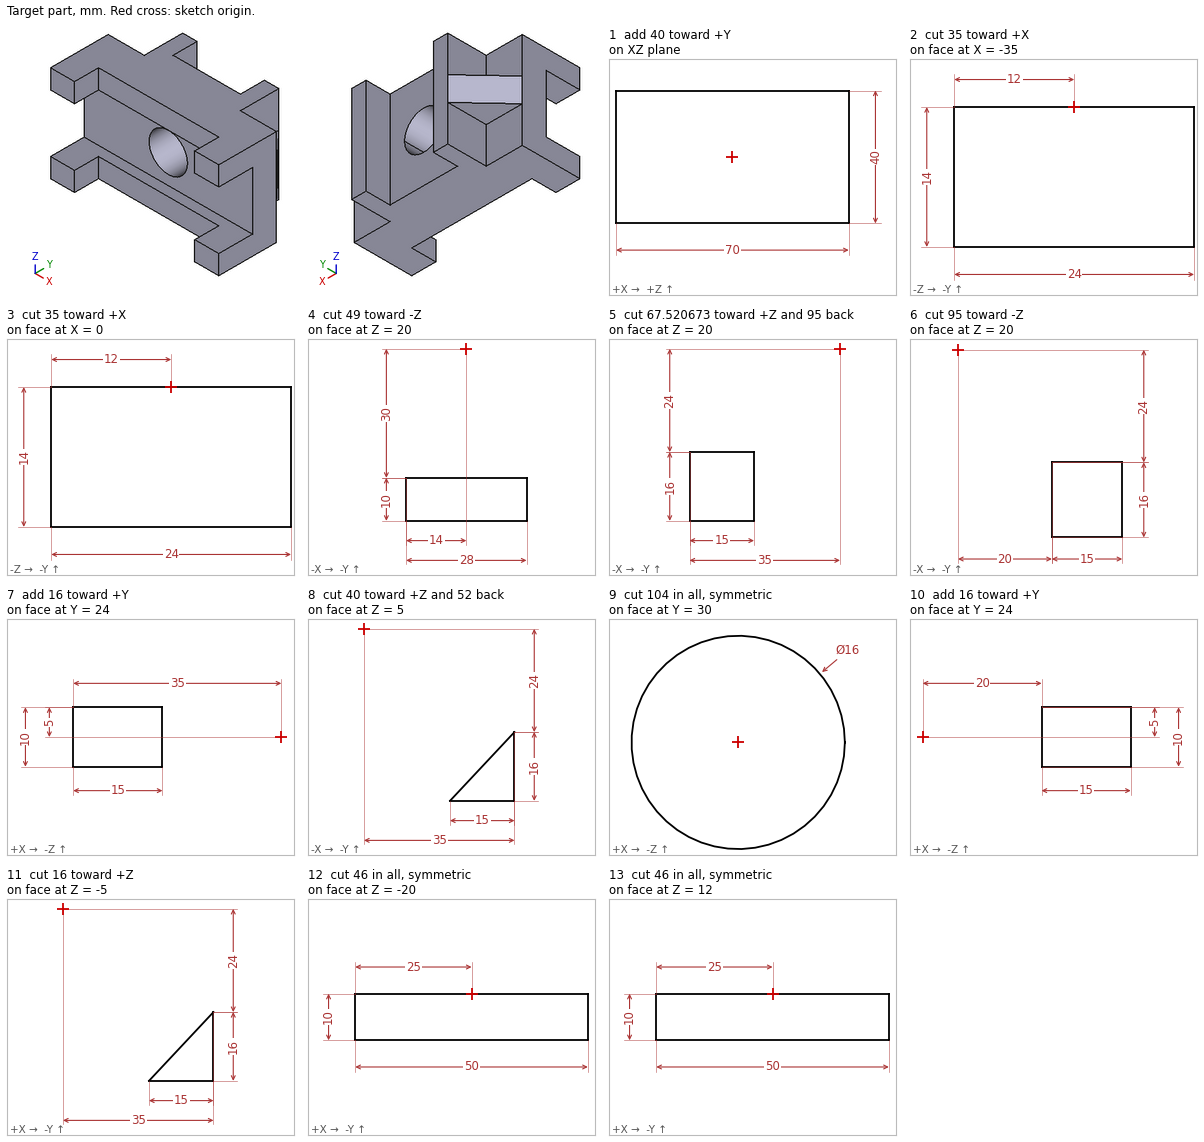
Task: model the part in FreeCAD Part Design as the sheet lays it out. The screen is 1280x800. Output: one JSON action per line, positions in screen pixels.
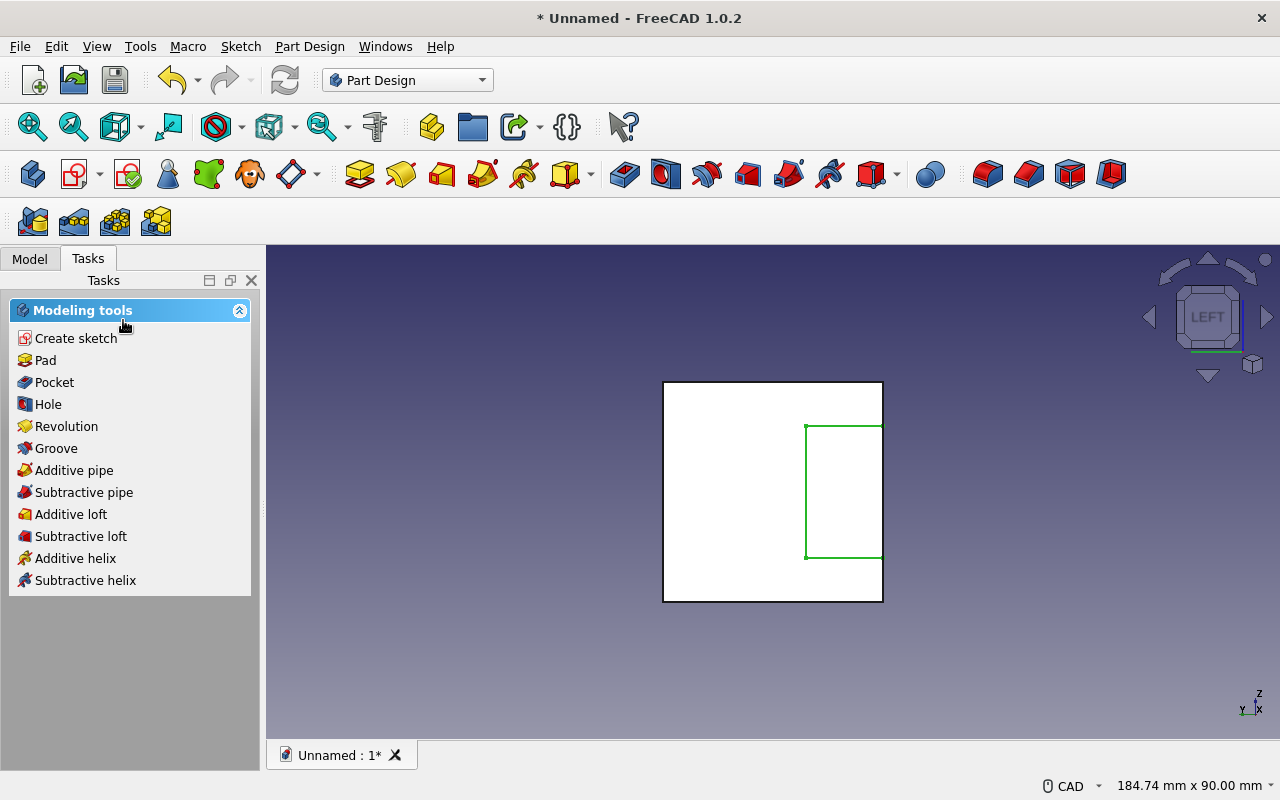
{"action": "left_click", "coordinate": [625, 174]}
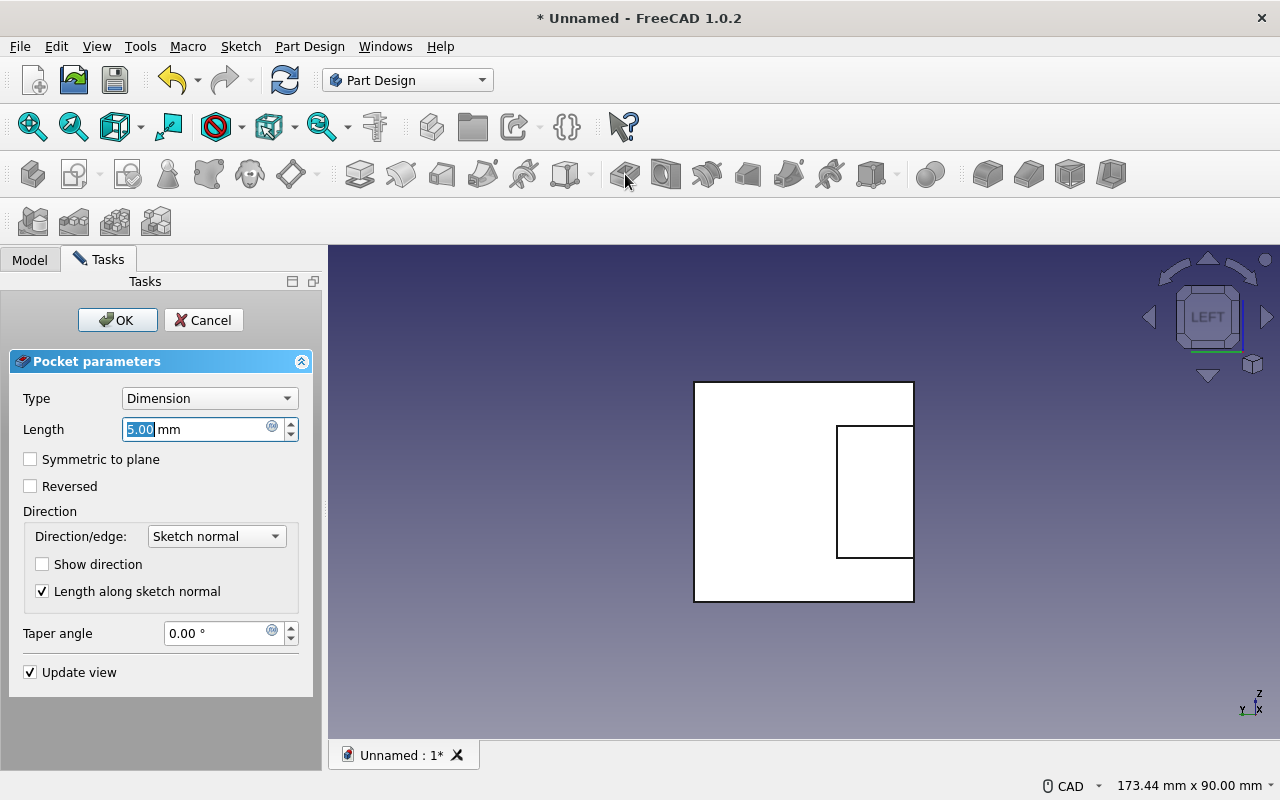
{"action": "type", "text": "35"}
{"action": "key", "text": "Tab"}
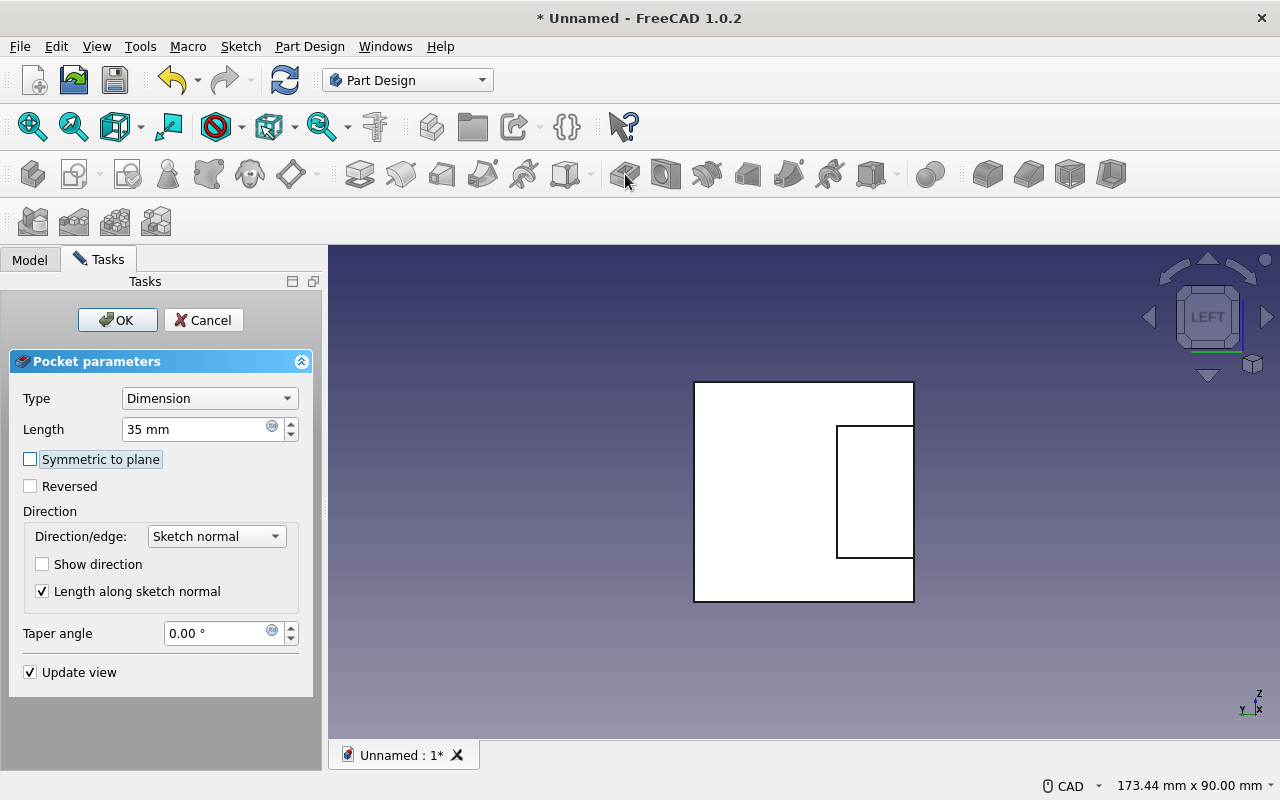
{"action": "left_click", "coordinate": [118, 320]}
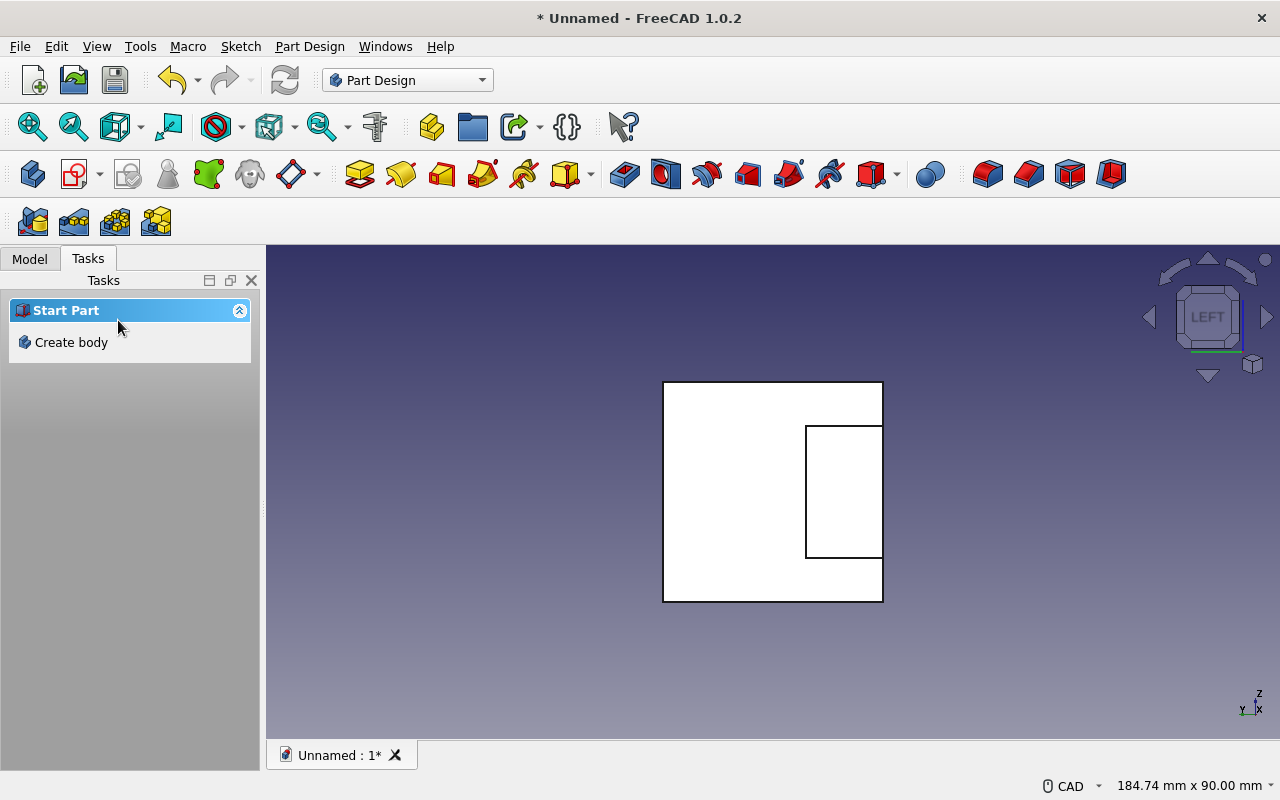
{"action": "key", "text": "v f"}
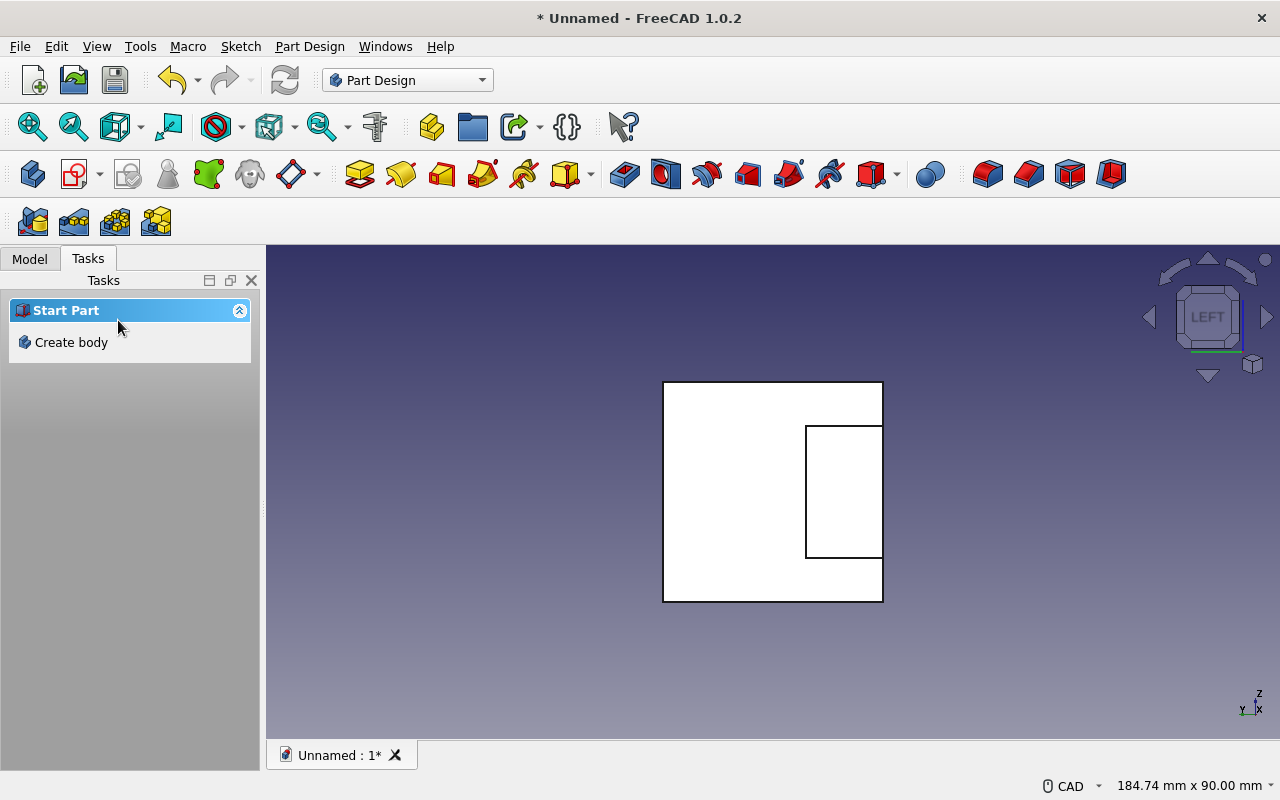
{"action": "left_click", "coordinate": [844, 472]}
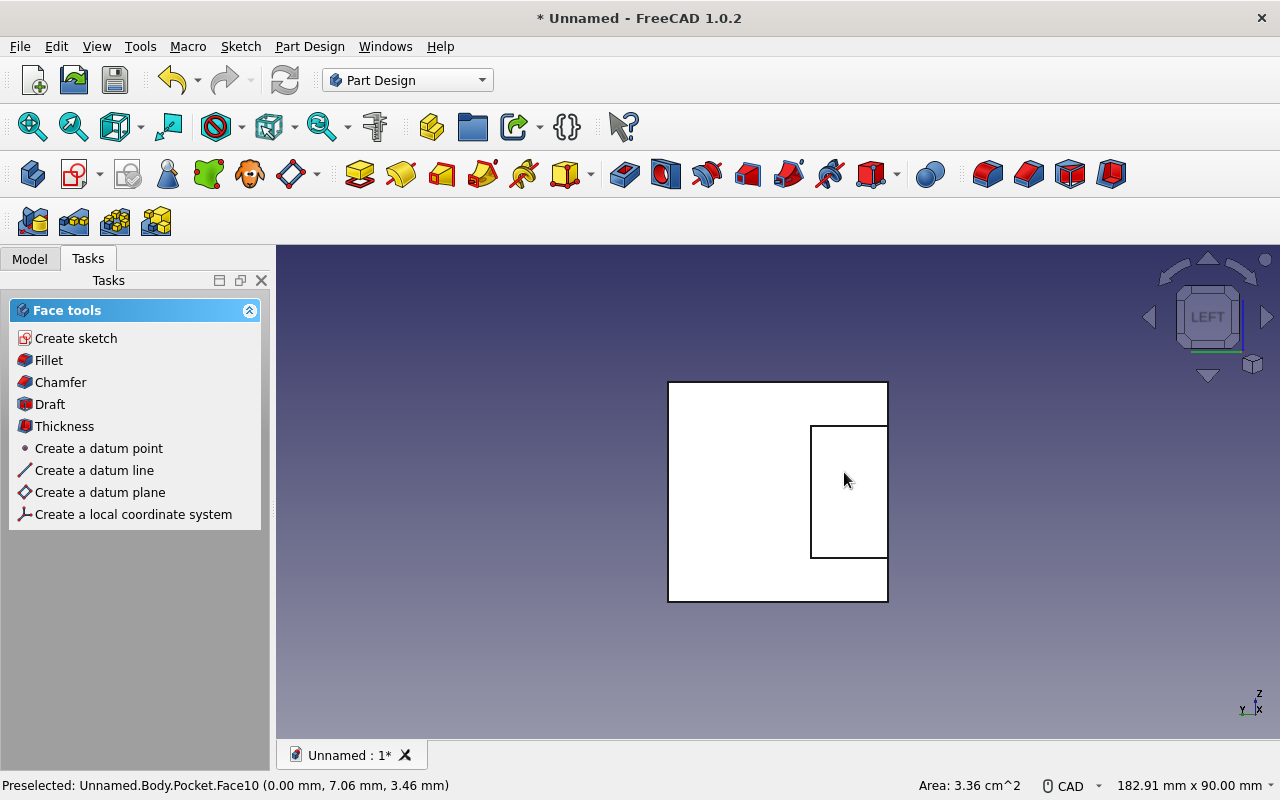
{"action": "left_click", "coordinate": [74, 174]}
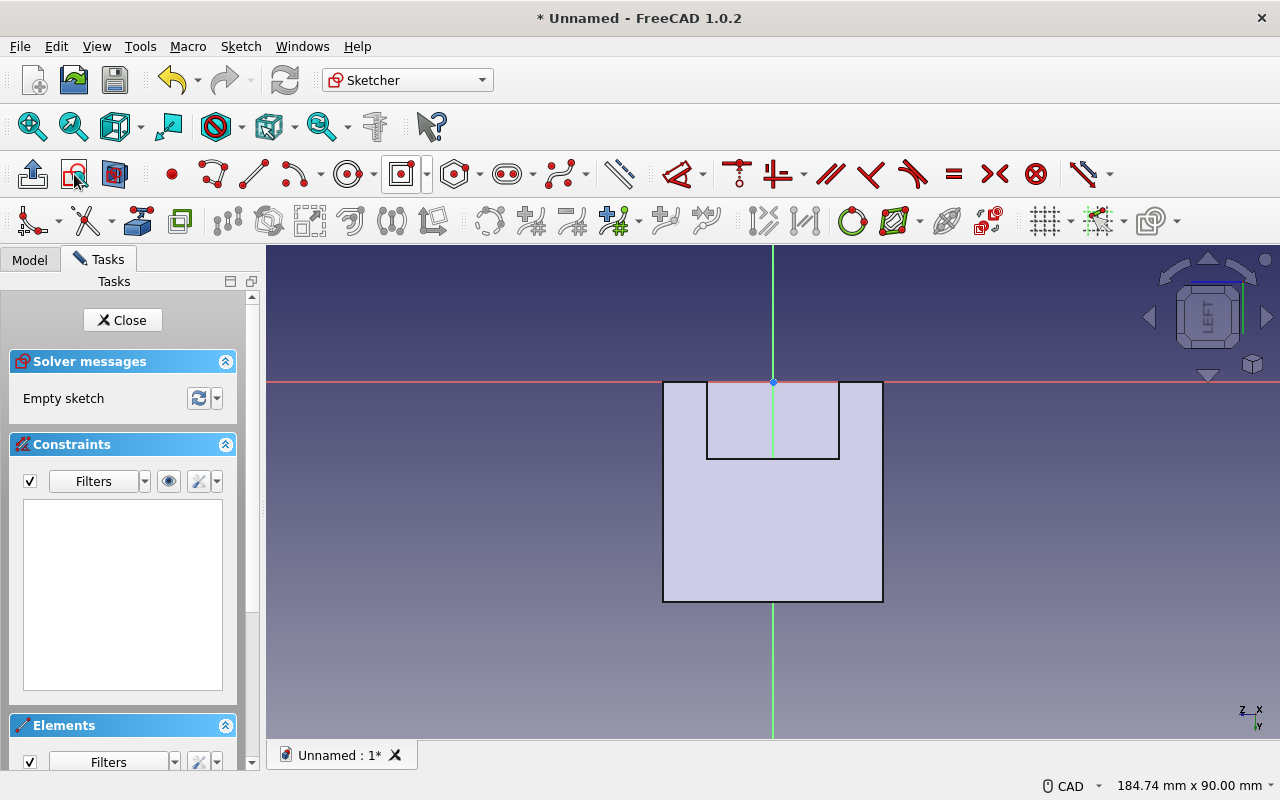
{"action": "left_click", "coordinate": [115, 174]}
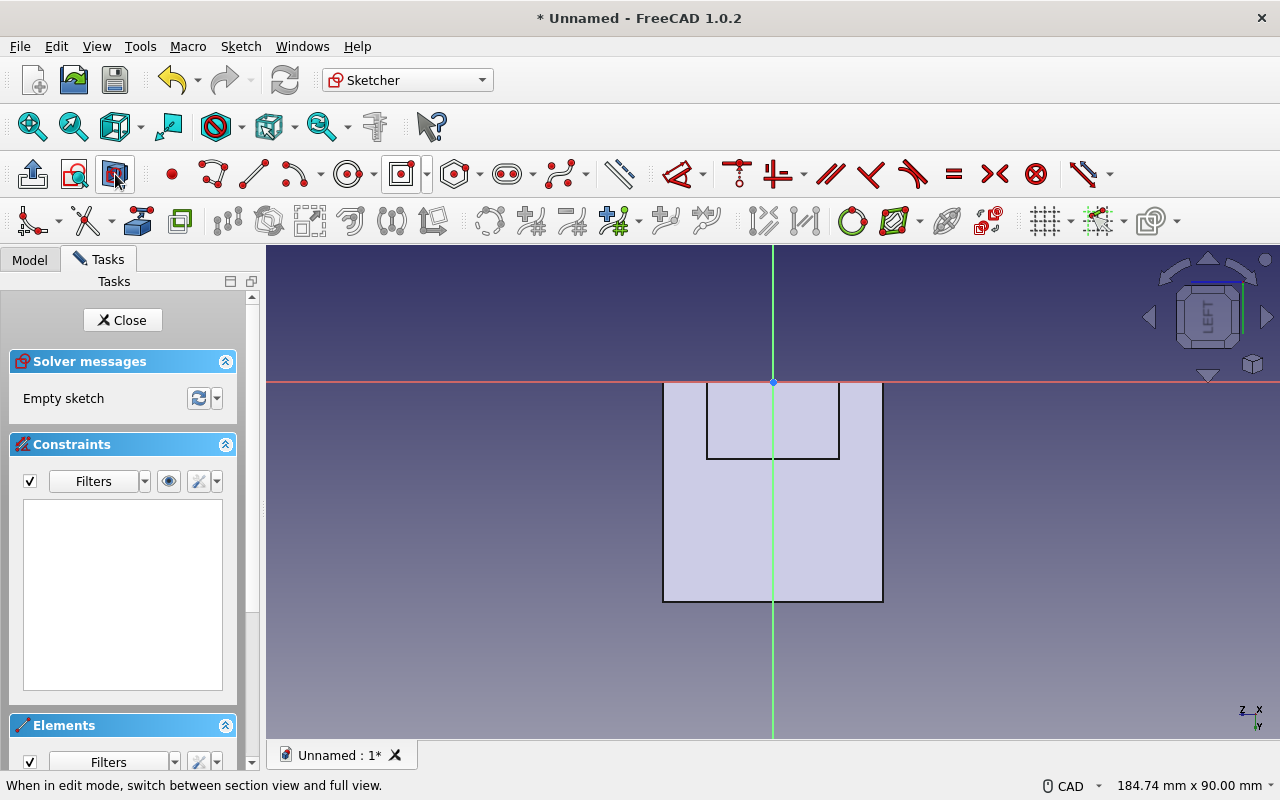
{"action": "scroll", "coordinate": [795, 397], "scroll_direction": "up", "scroll_amount": 7}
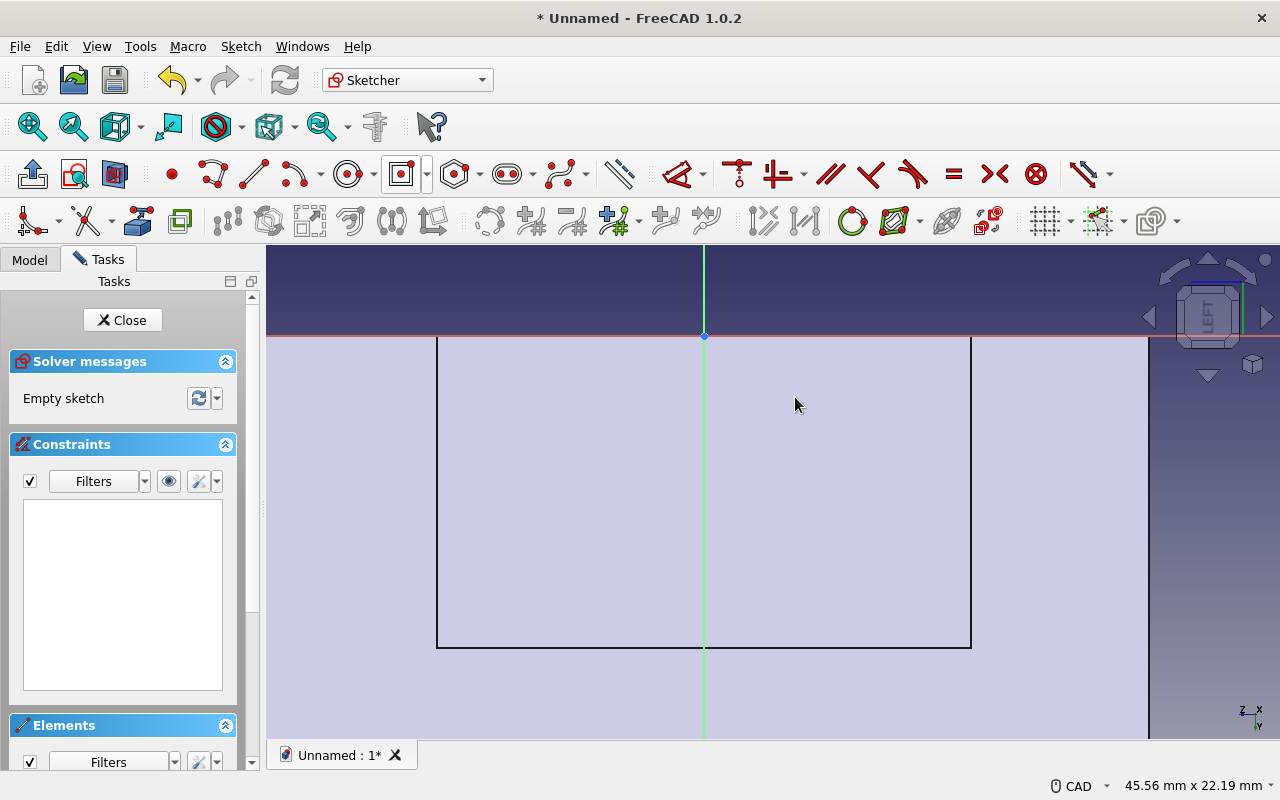
{"action": "key", "text": "g r"}